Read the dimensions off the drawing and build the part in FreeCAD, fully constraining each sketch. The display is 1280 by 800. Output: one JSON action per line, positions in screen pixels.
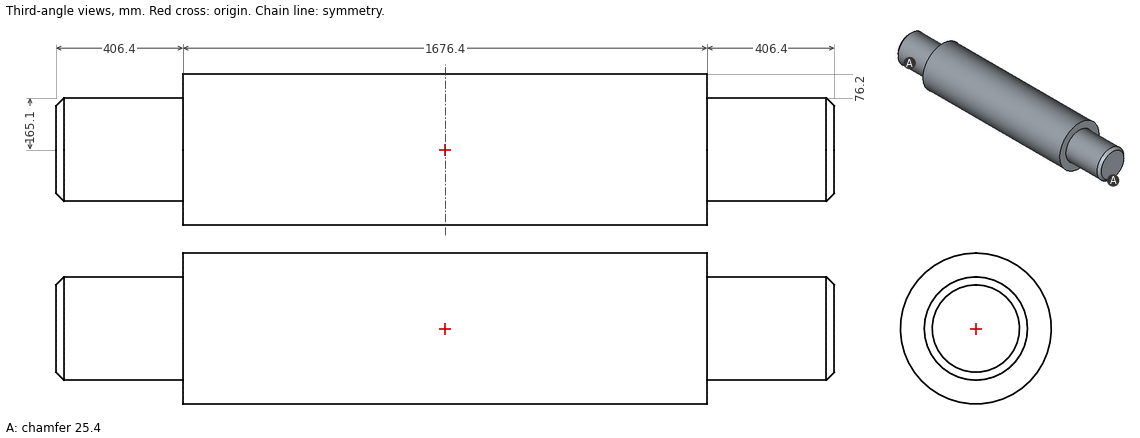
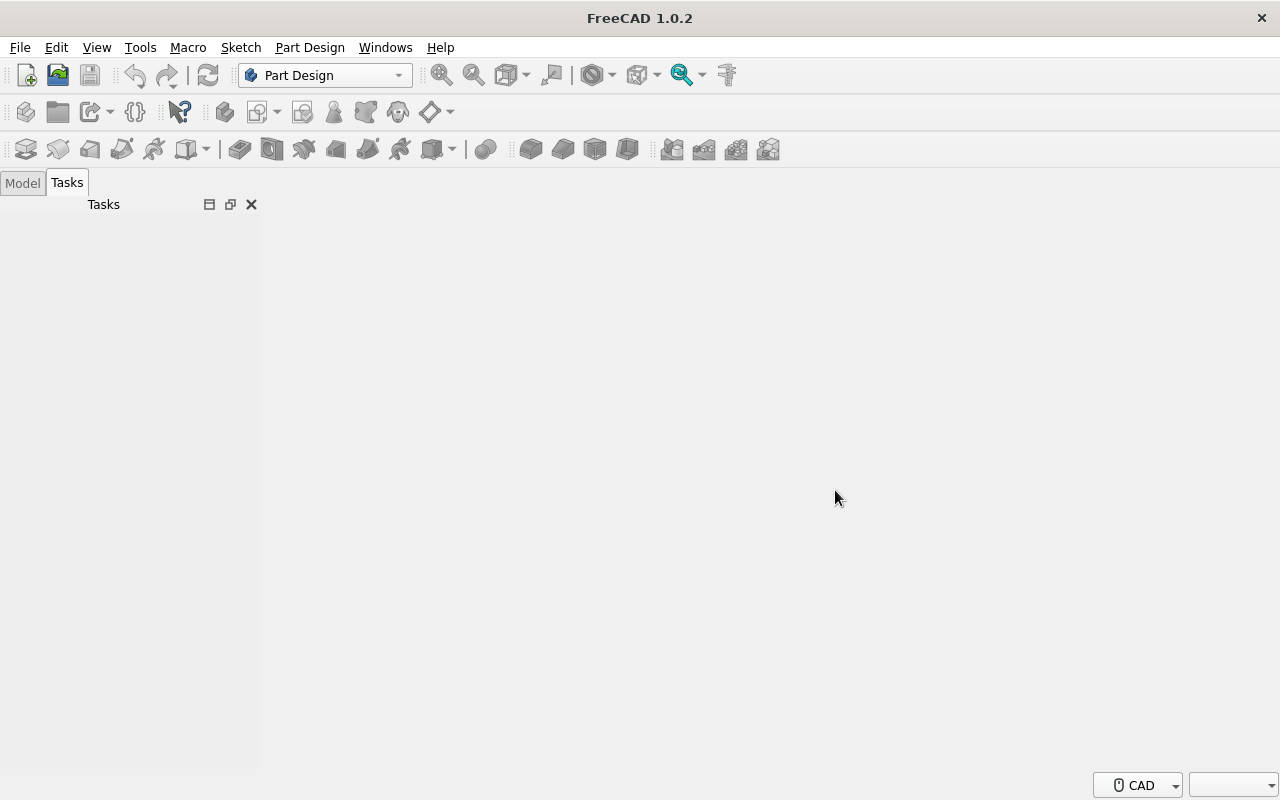
{"action": "key", "text": "ctrl+n"}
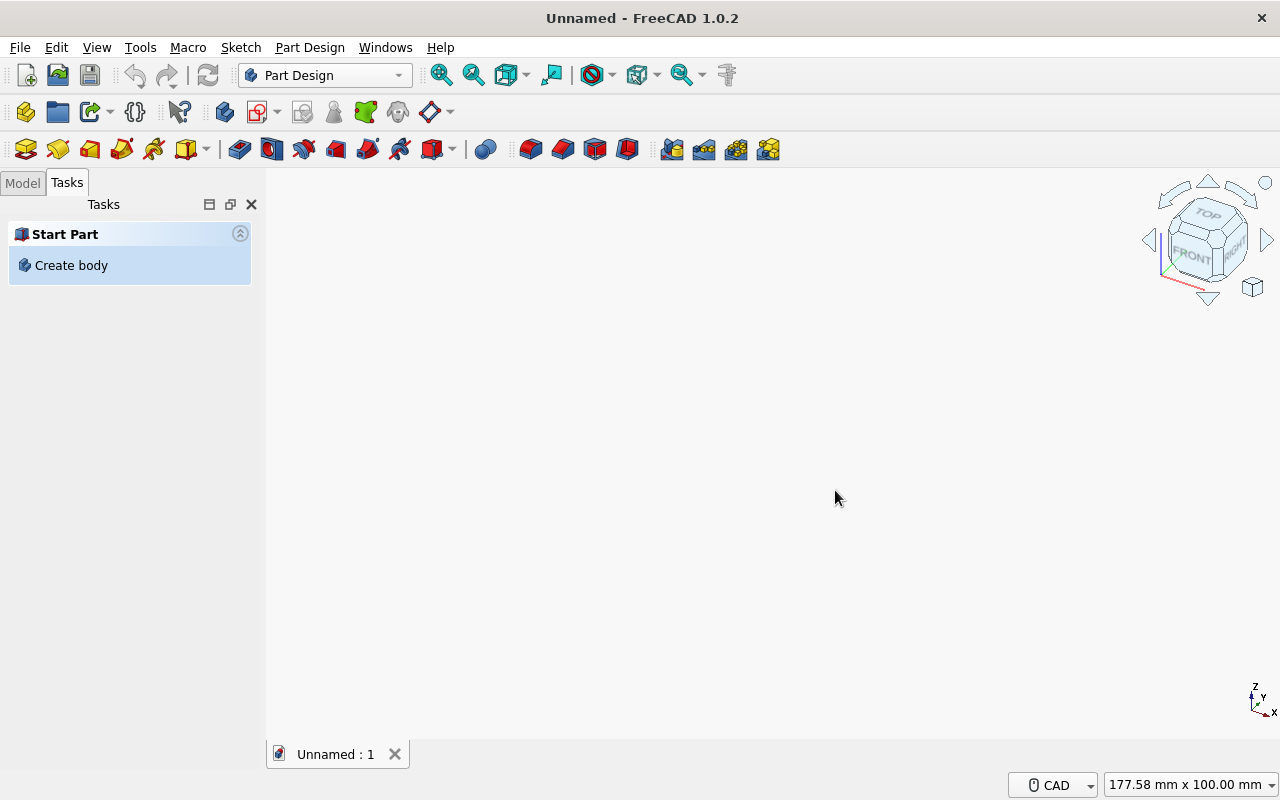
{"action": "left_click", "coordinate": [258, 112]}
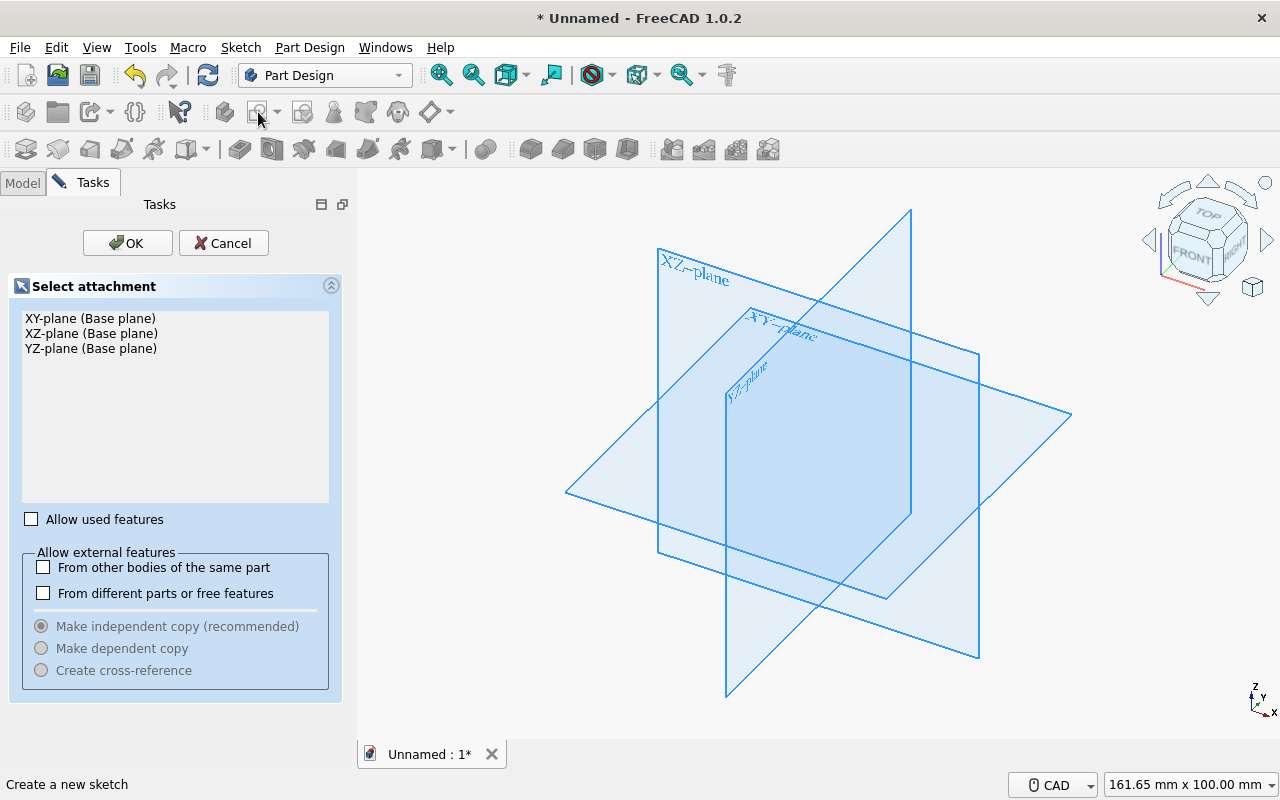
{"action": "left_click", "coordinate": [82, 318]}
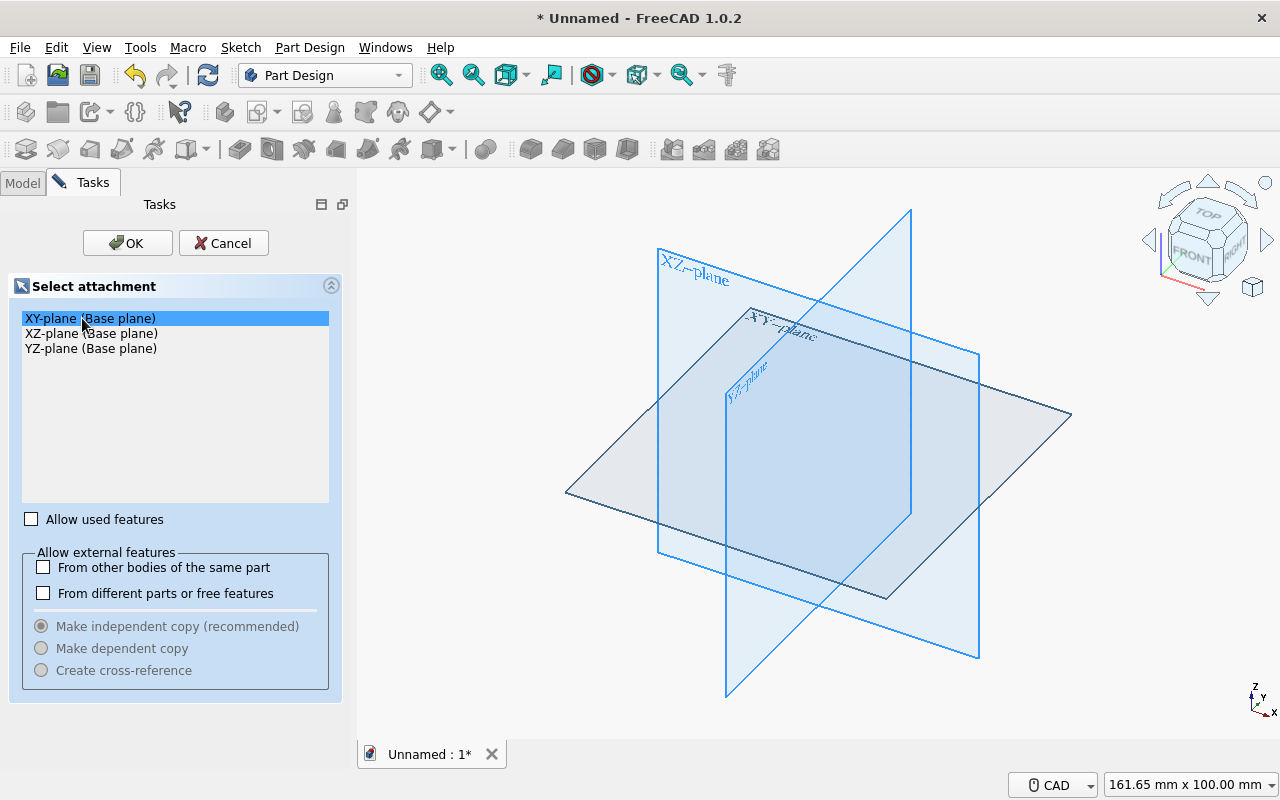
{"action": "left_click", "coordinate": [128, 243]}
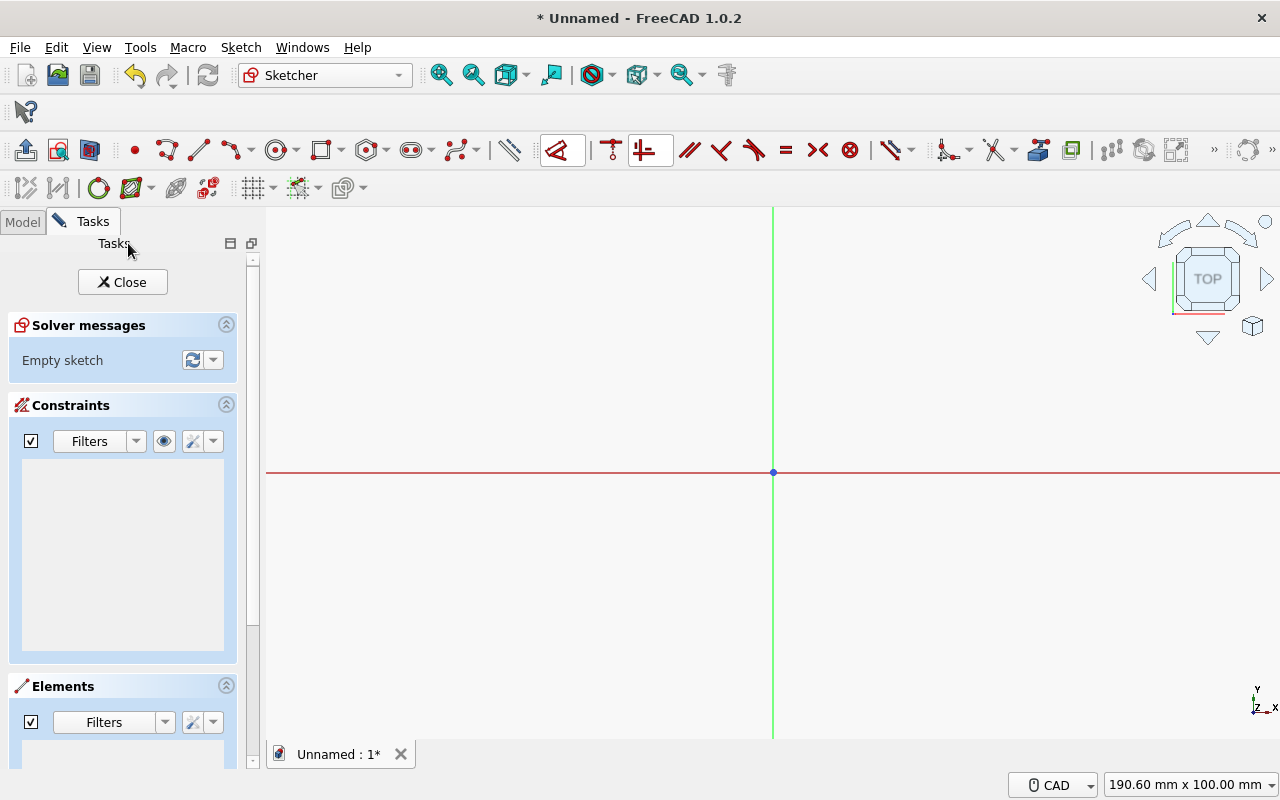
{"action": "scroll", "coordinate": [701, 507], "scroll_direction": "down", "scroll_amount": 15}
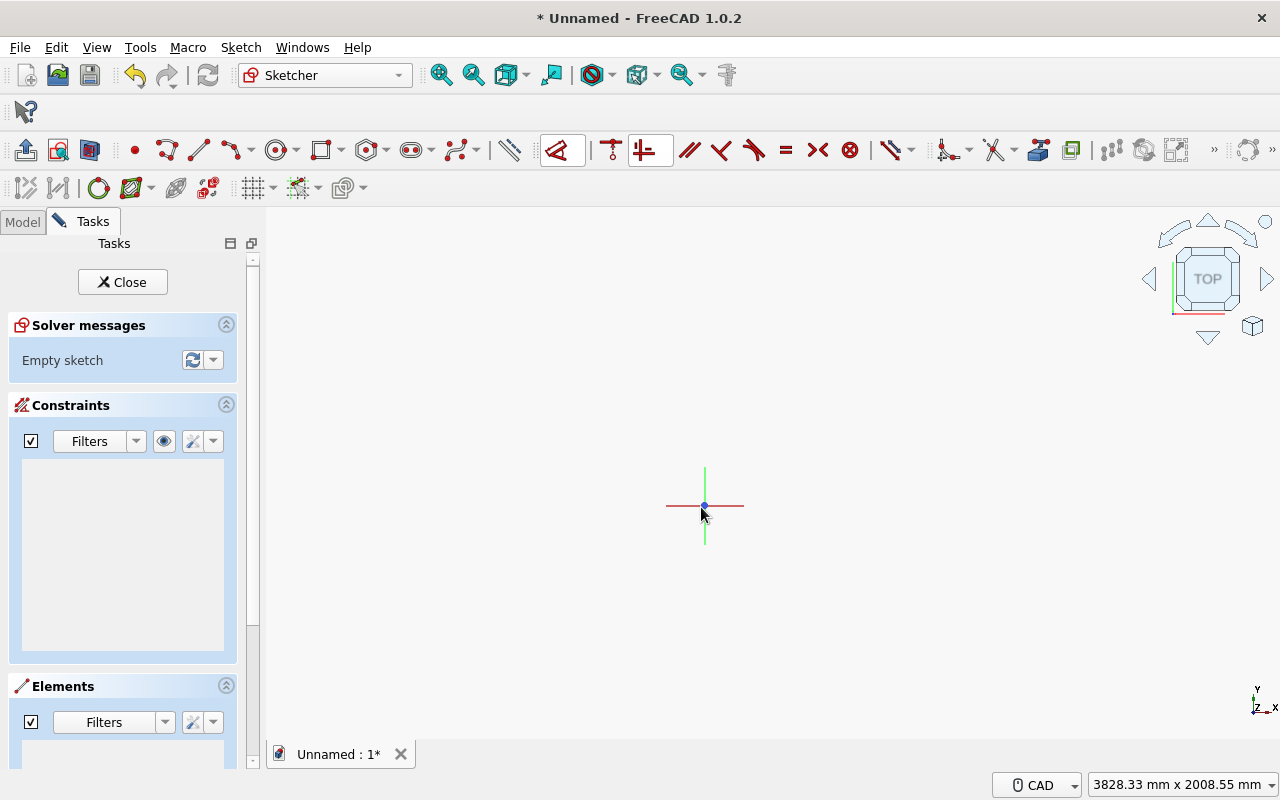
{"action": "left_click", "coordinate": [168, 150]}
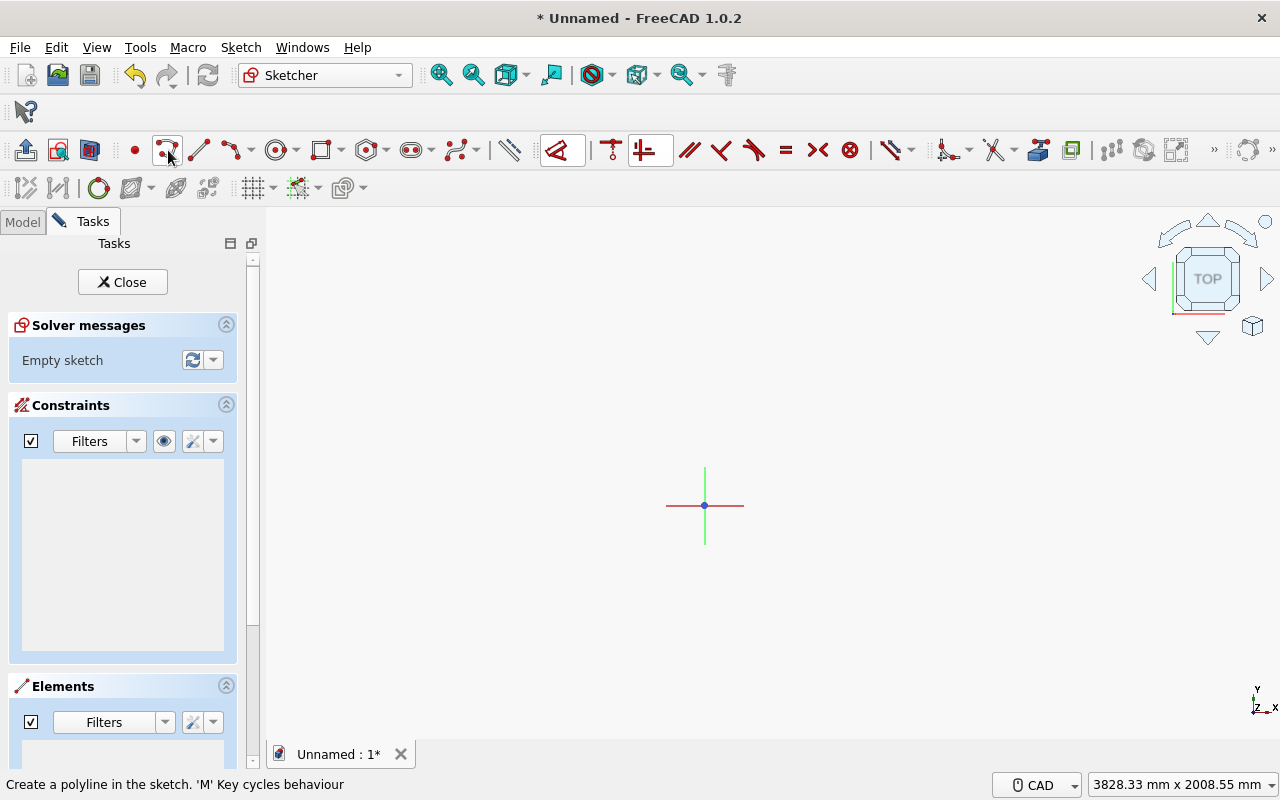
{"action": "left_click", "coordinate": [927, 462]}
{"action": "left_click", "coordinate": [927, 442]}
{"action": "left_click", "coordinate": [483, 442]}
{"action": "left_click", "coordinate": [483, 462]}
{"action": "left_click", "coordinate": [375, 462]}
{"action": "left_click", "coordinate": [375, 506]}
{"action": "left_click", "coordinate": [1035, 497]}
{"action": "left_click", "coordinate": [1035, 462]}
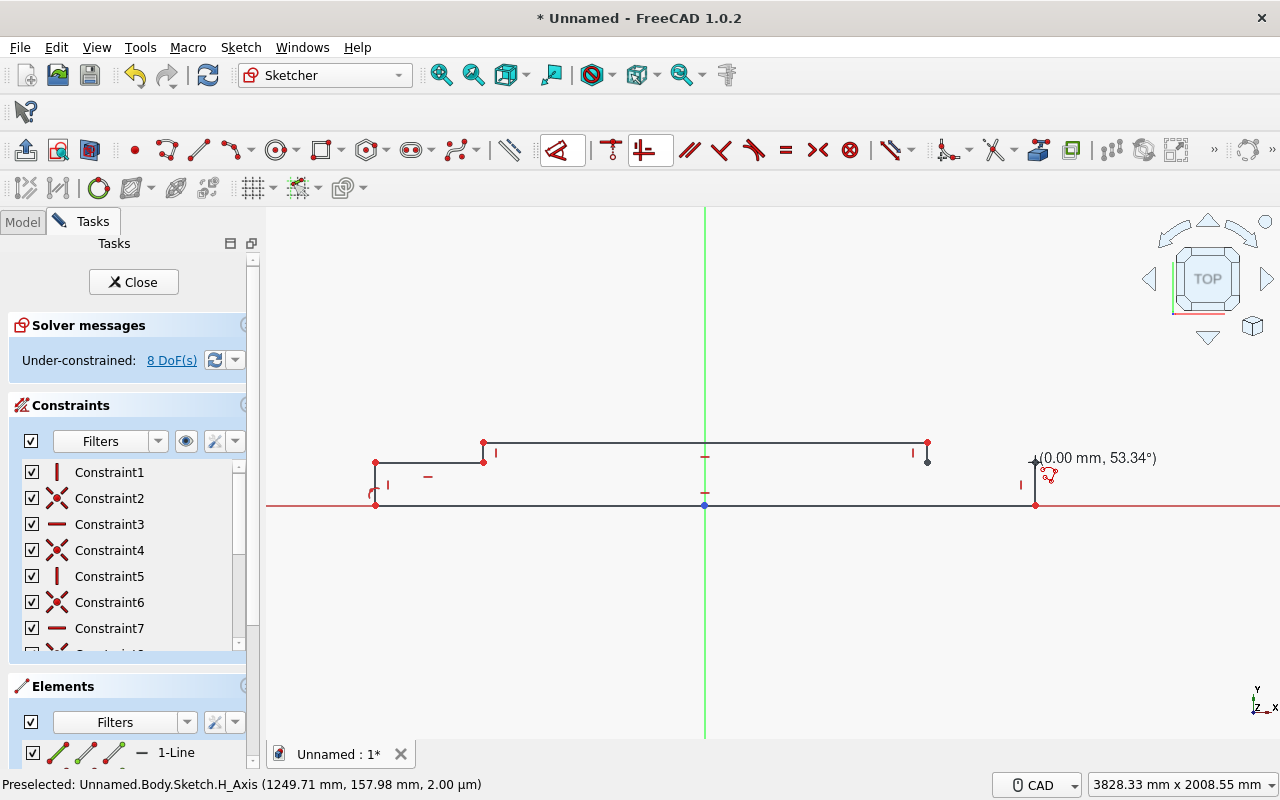
{"action": "scroll", "coordinate": [927, 462], "scroll_direction": "up", "scroll_amount": 3}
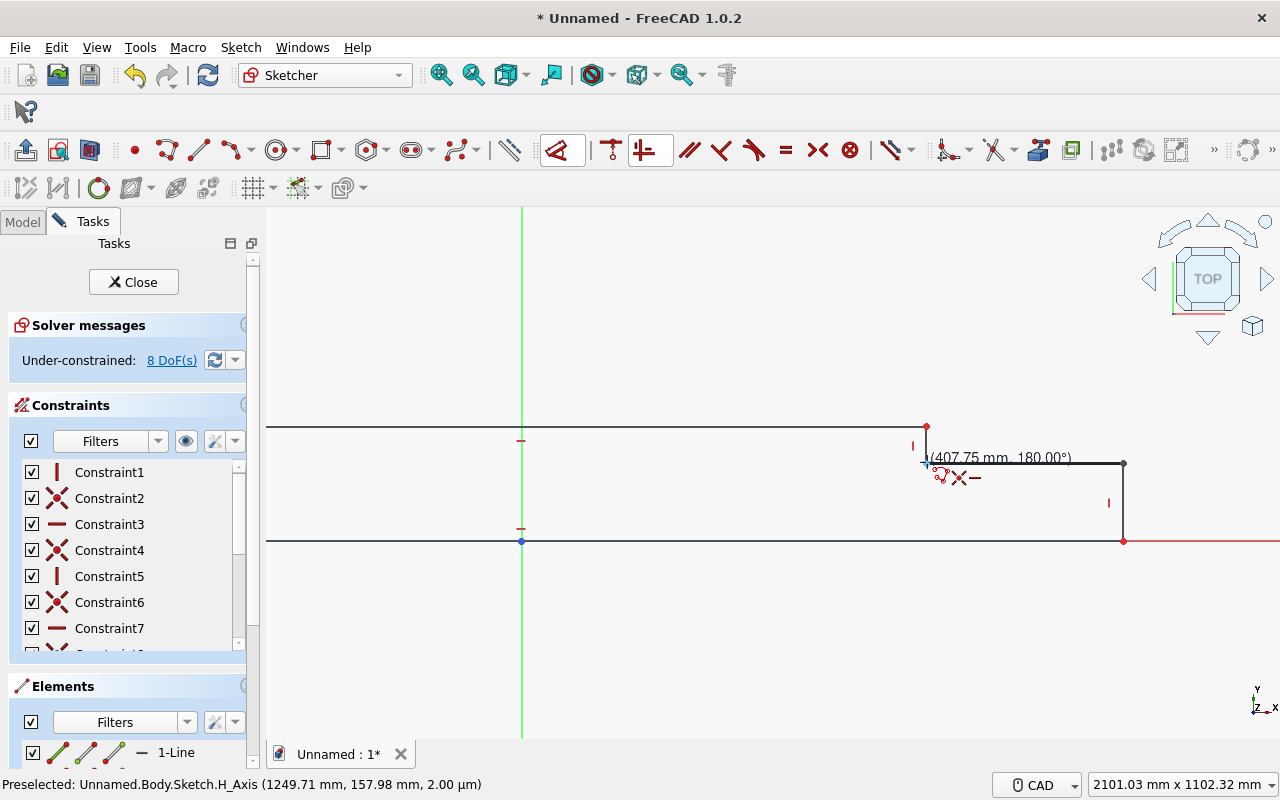
{"action": "left_click", "coordinate": [926, 463]}
{"action": "key", "text": "Escape"}
{"action": "key", "text": "Escape"}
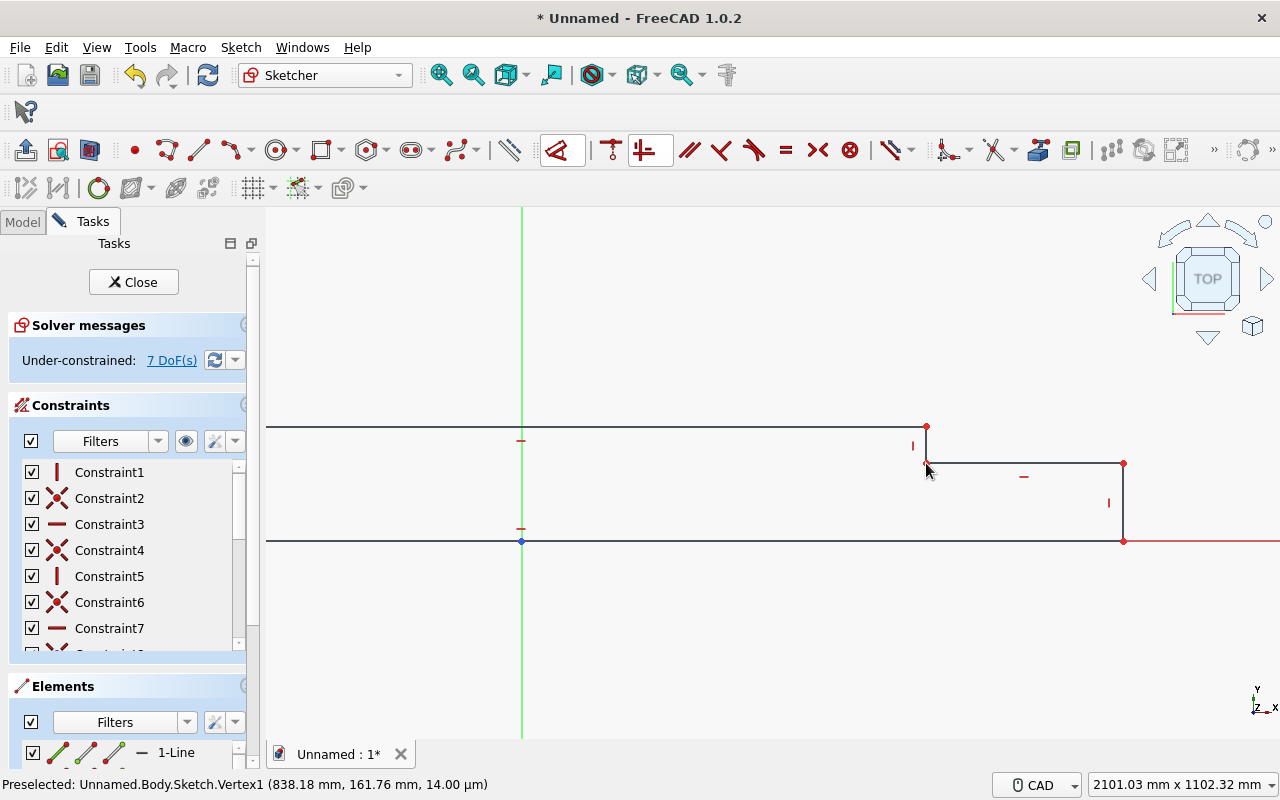
{"action": "left_click", "coordinate": [926, 463]}